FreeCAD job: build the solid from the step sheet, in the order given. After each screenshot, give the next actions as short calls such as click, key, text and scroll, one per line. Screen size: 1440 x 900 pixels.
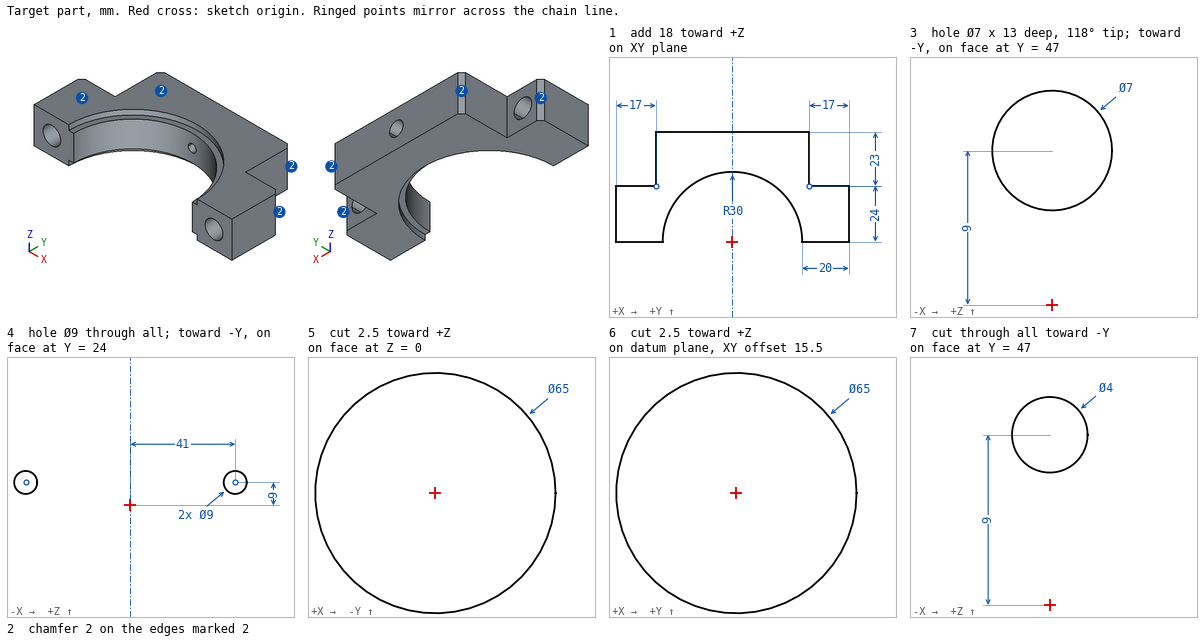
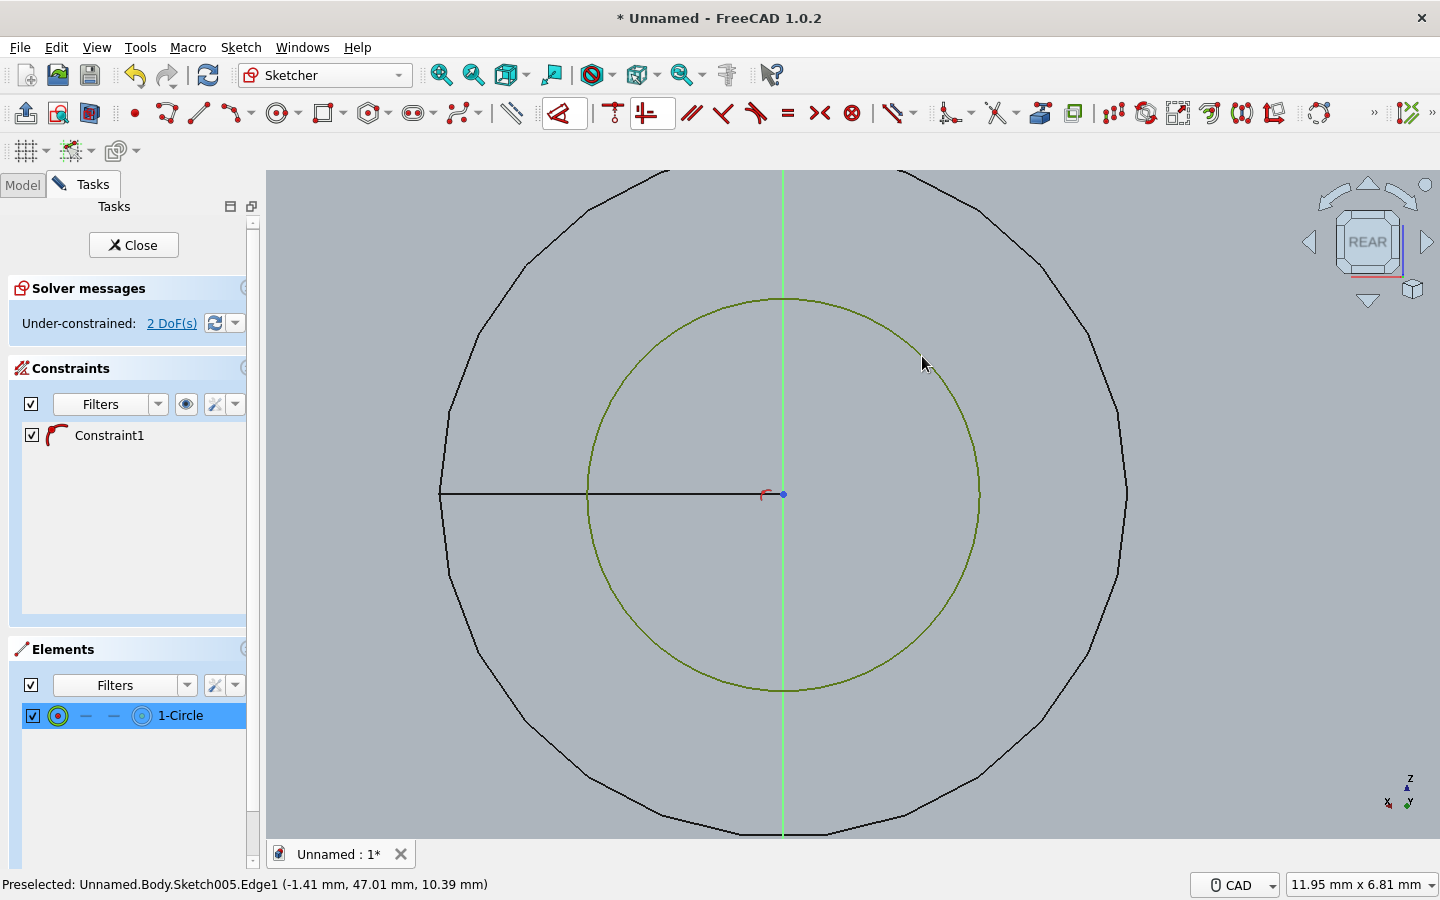
click(582, 114)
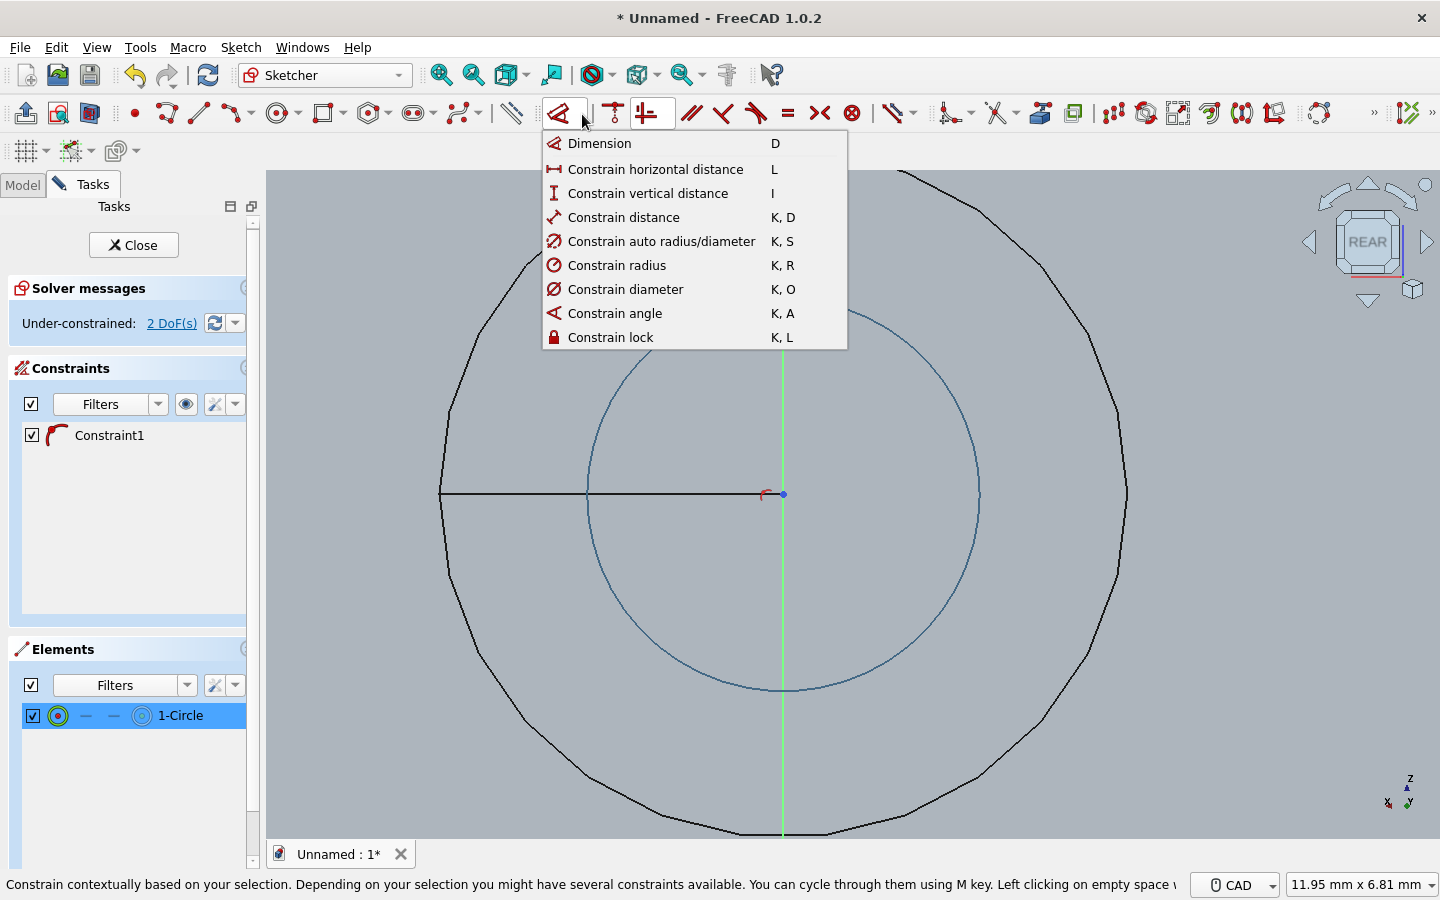
click(695, 289)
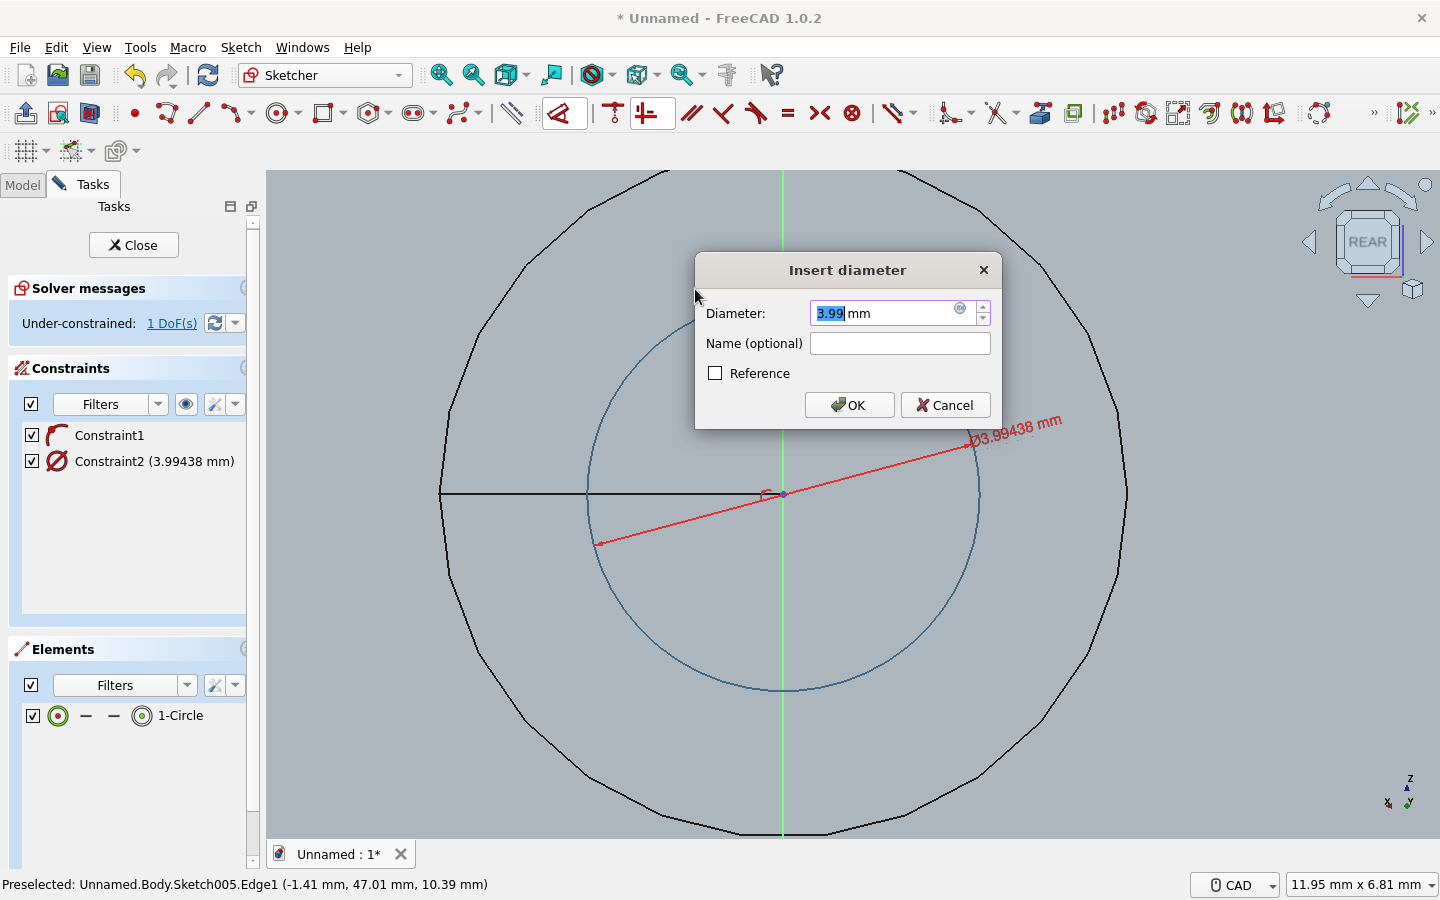
text(4)
key(Return)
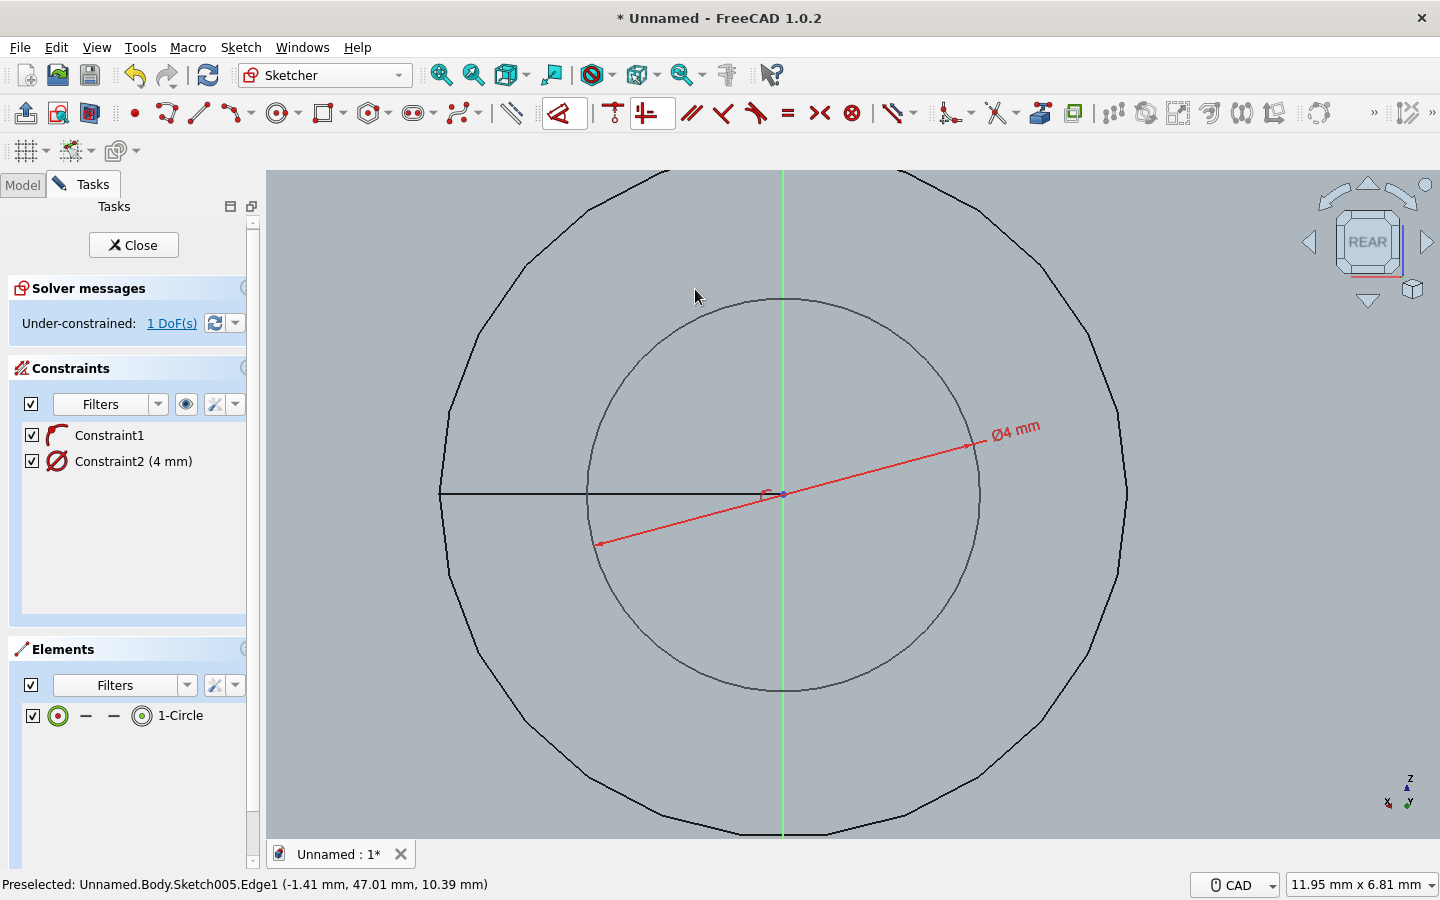
click(783, 495)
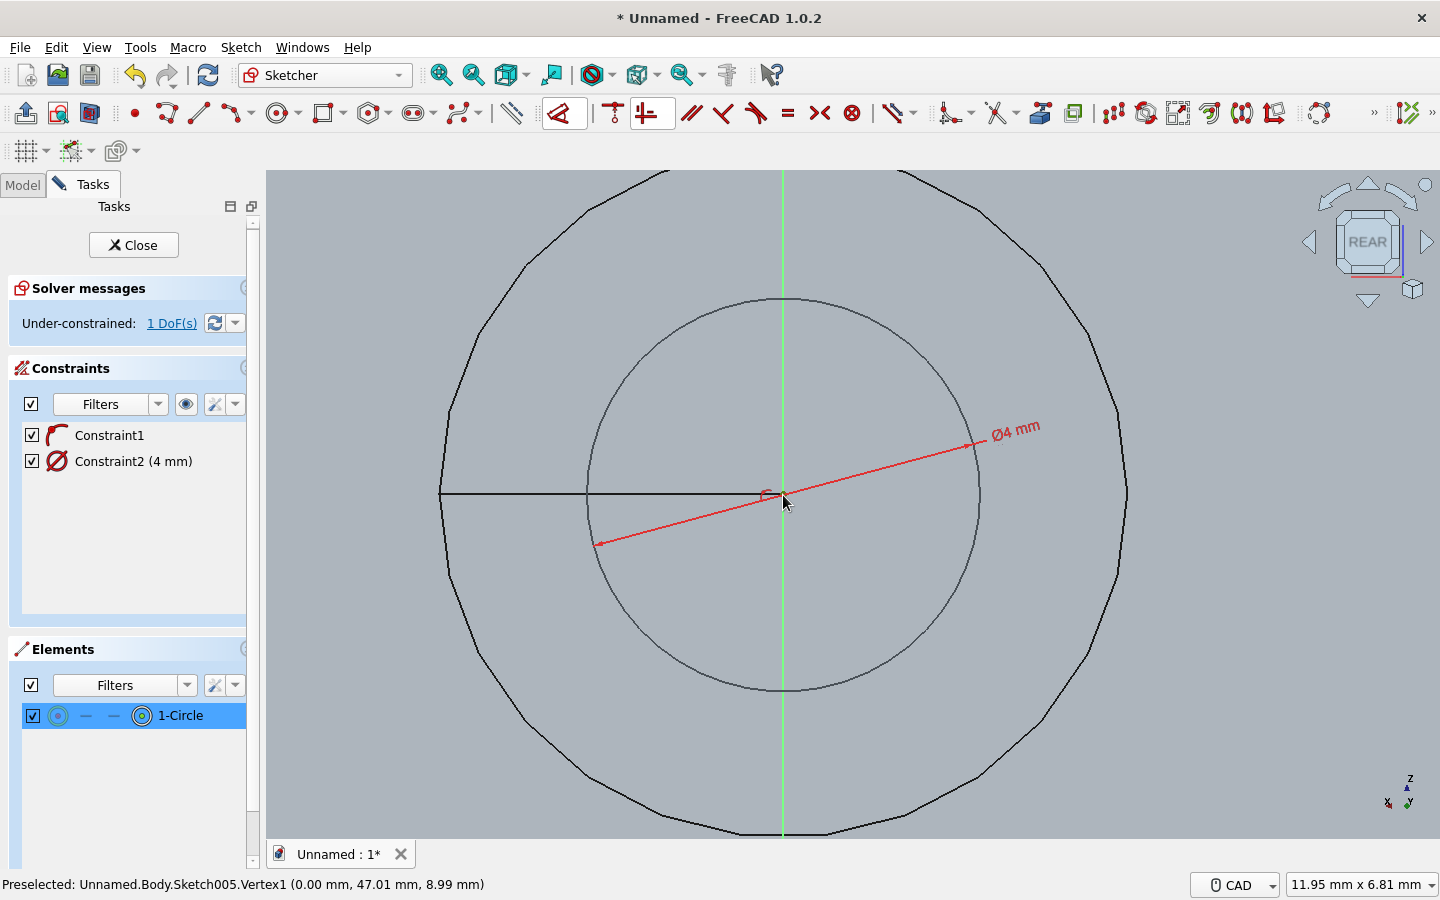
key(i)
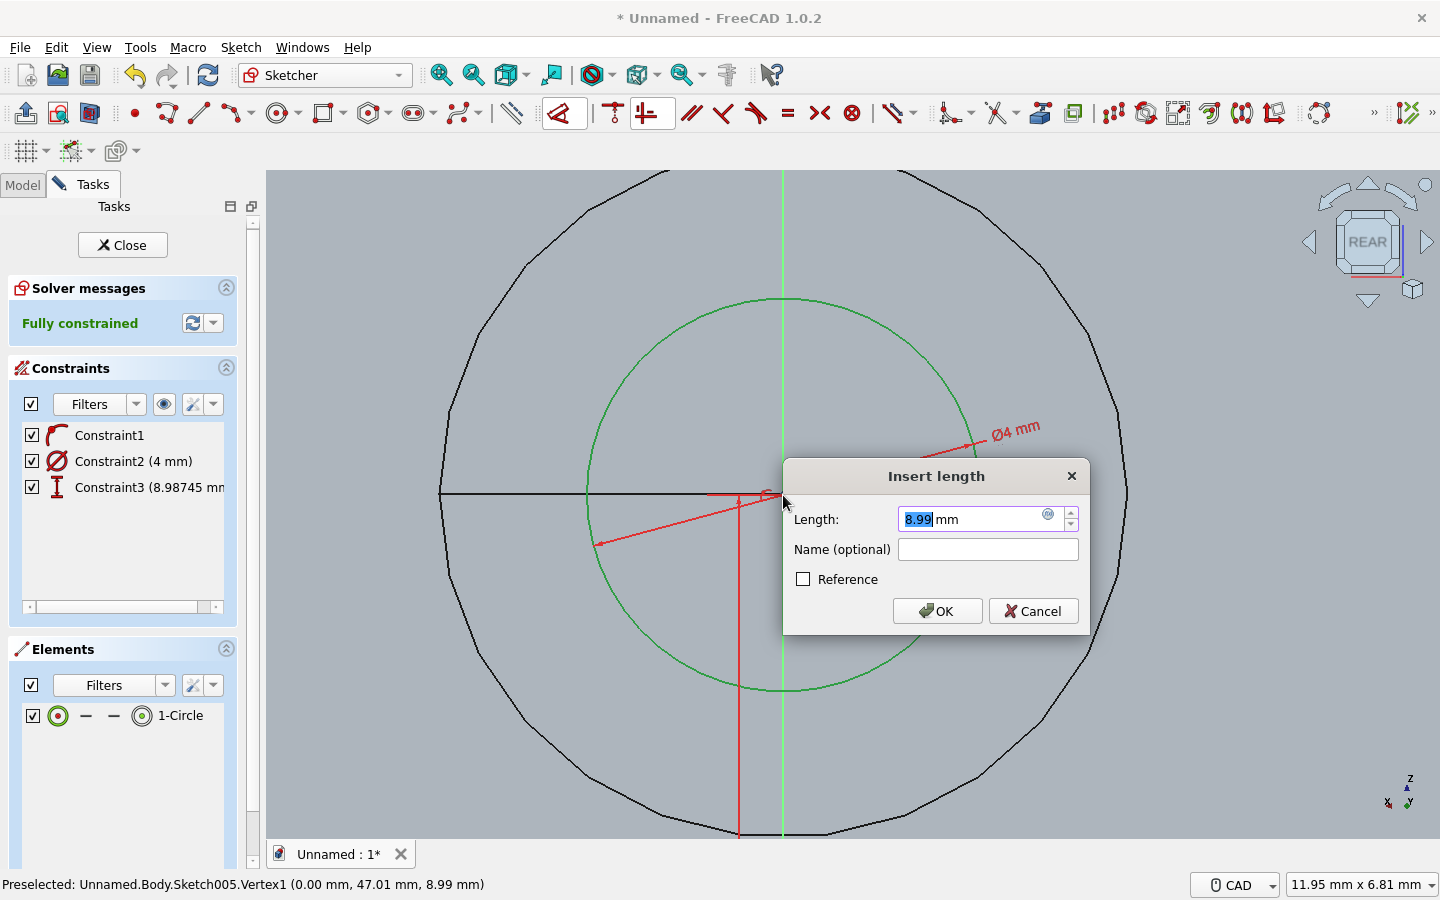
text(9)
key(Return)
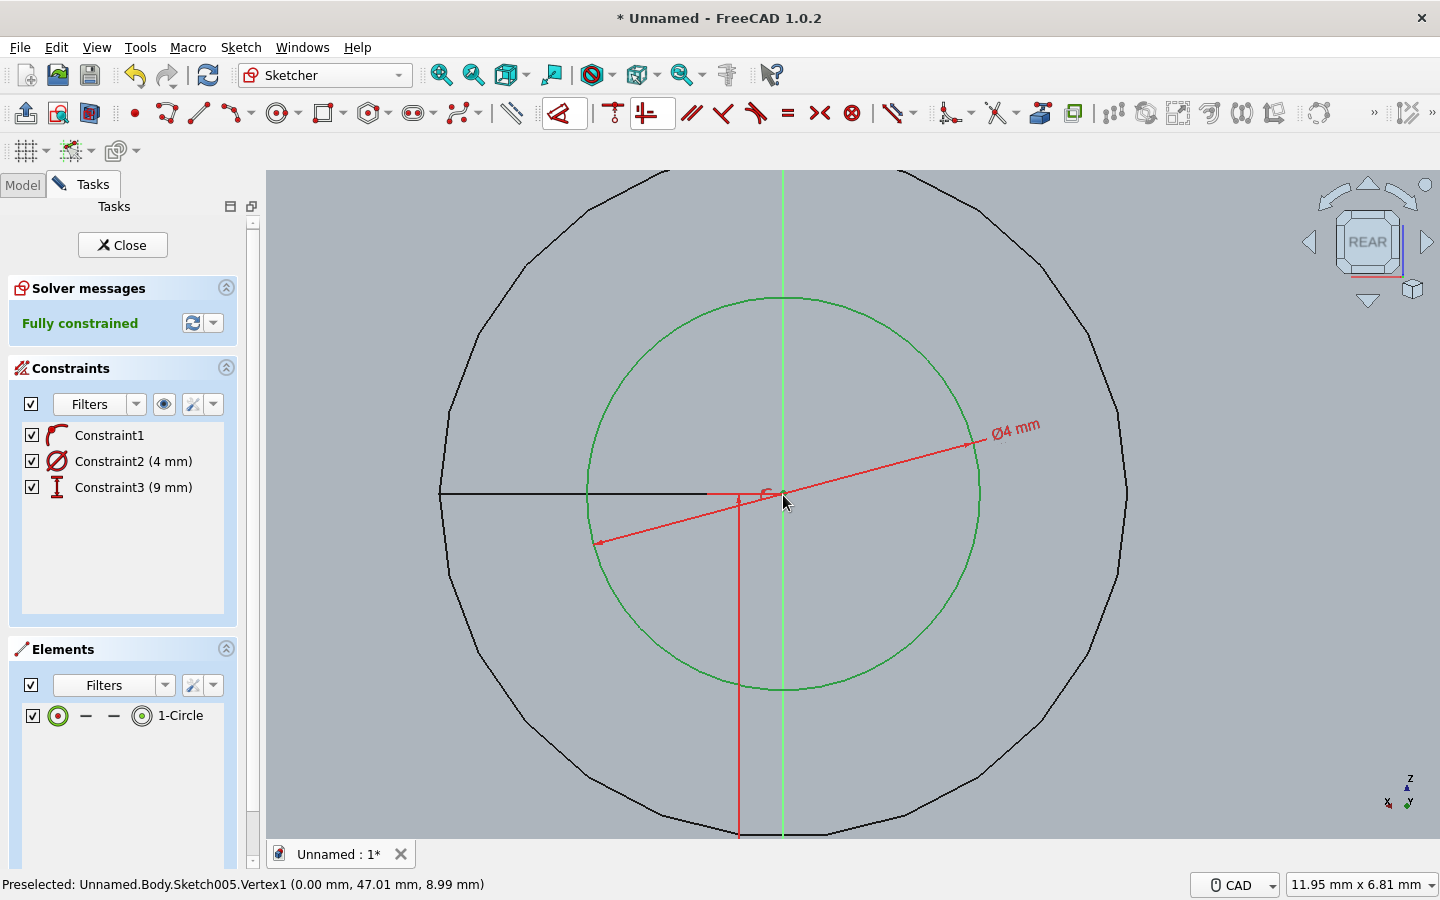
click(123, 245)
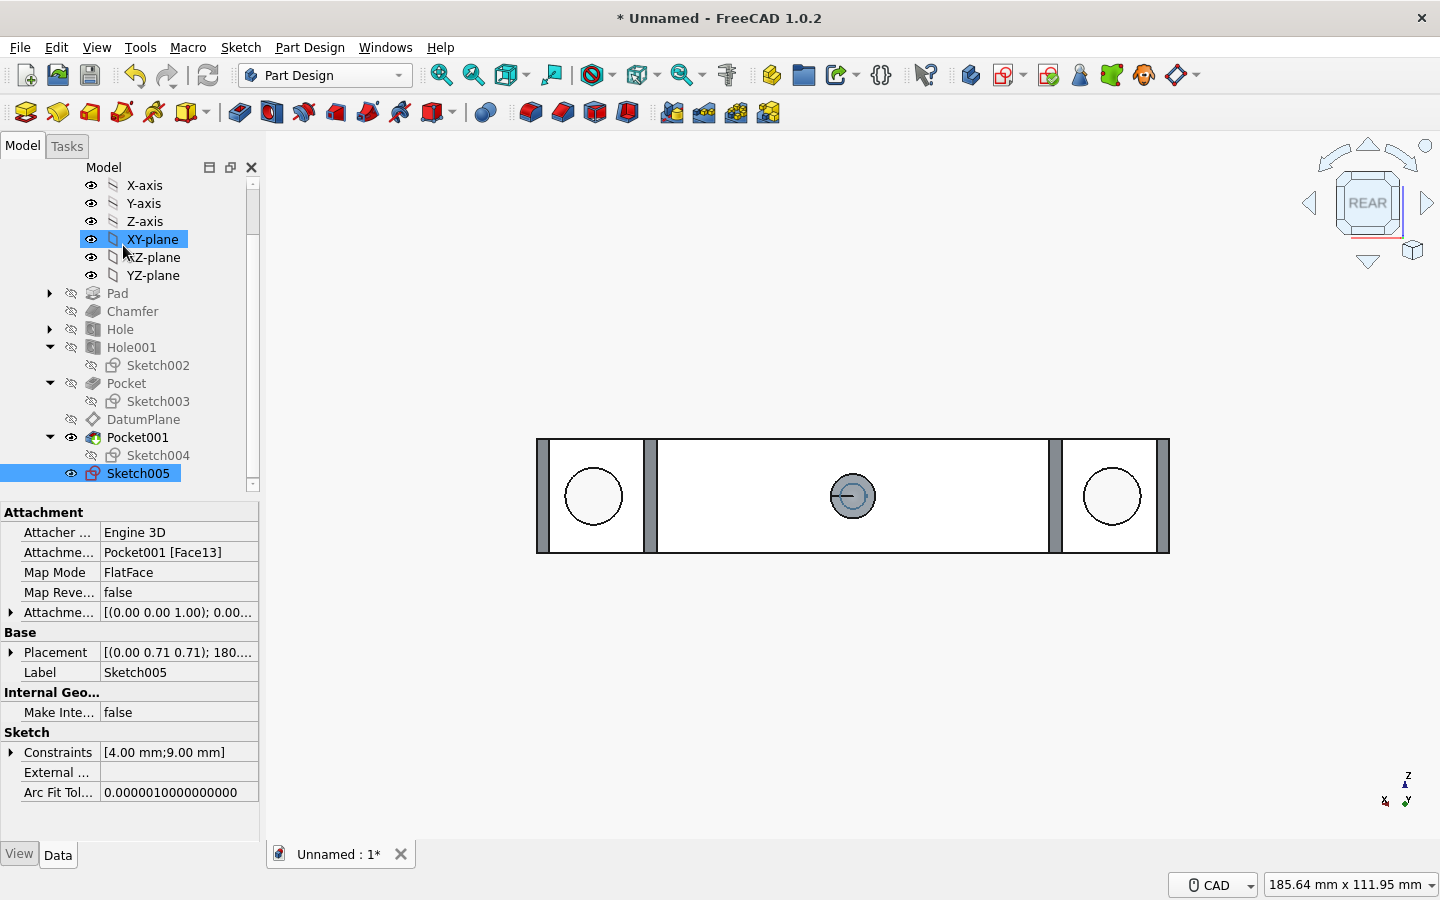
click(240, 112)